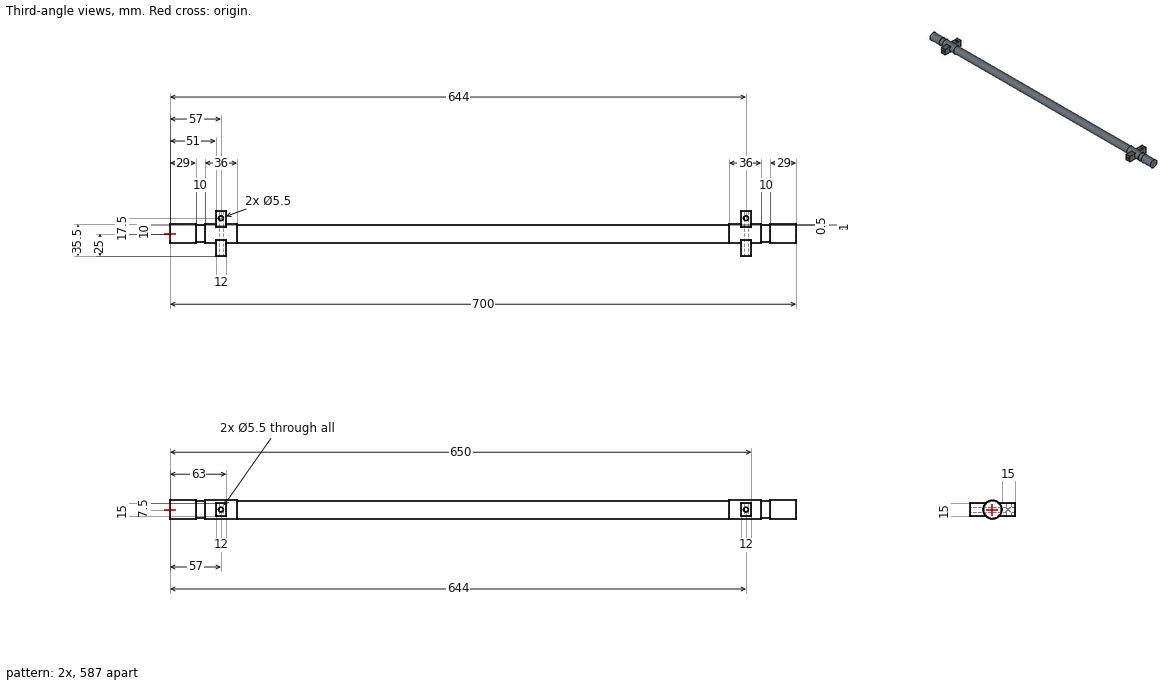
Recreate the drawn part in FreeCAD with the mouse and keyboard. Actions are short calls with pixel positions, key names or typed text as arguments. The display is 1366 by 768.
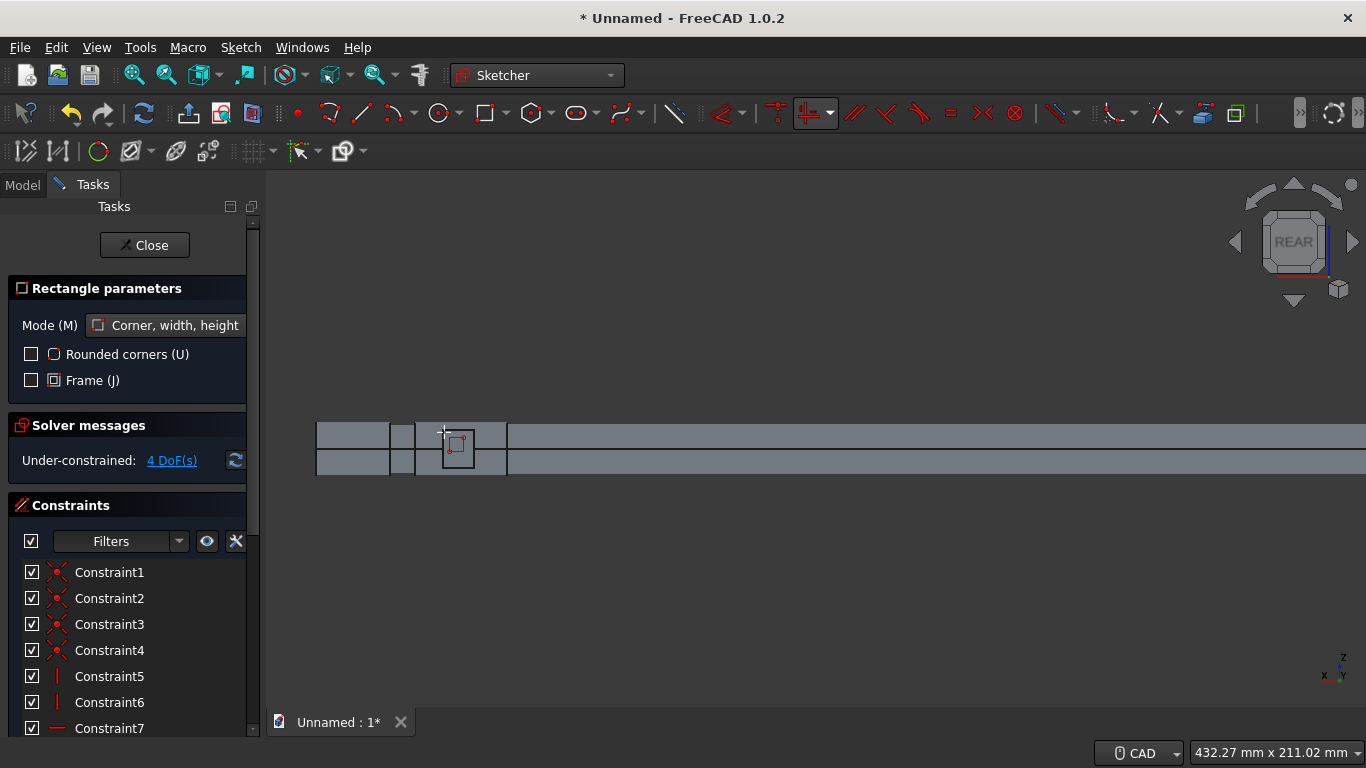
click(443, 430)
click(474, 468)
key(Escape)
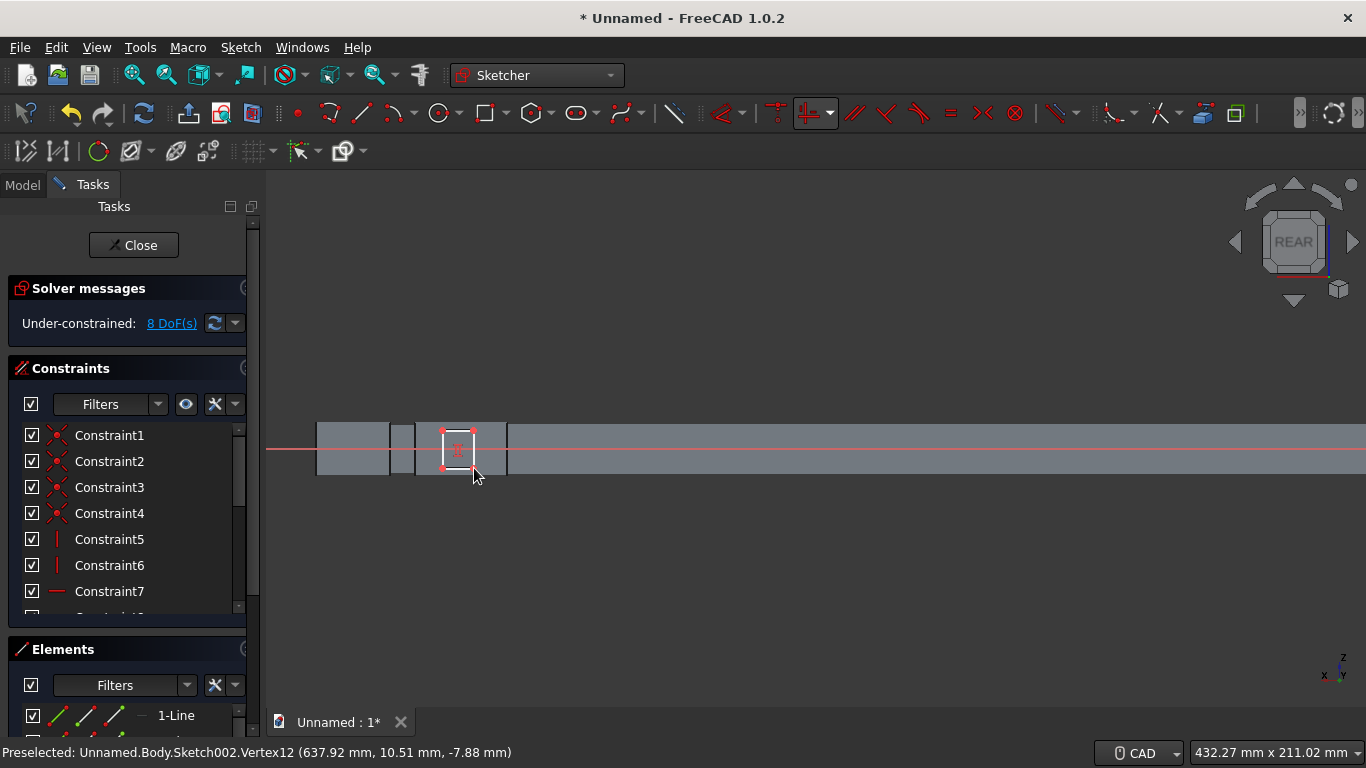
click(722, 114)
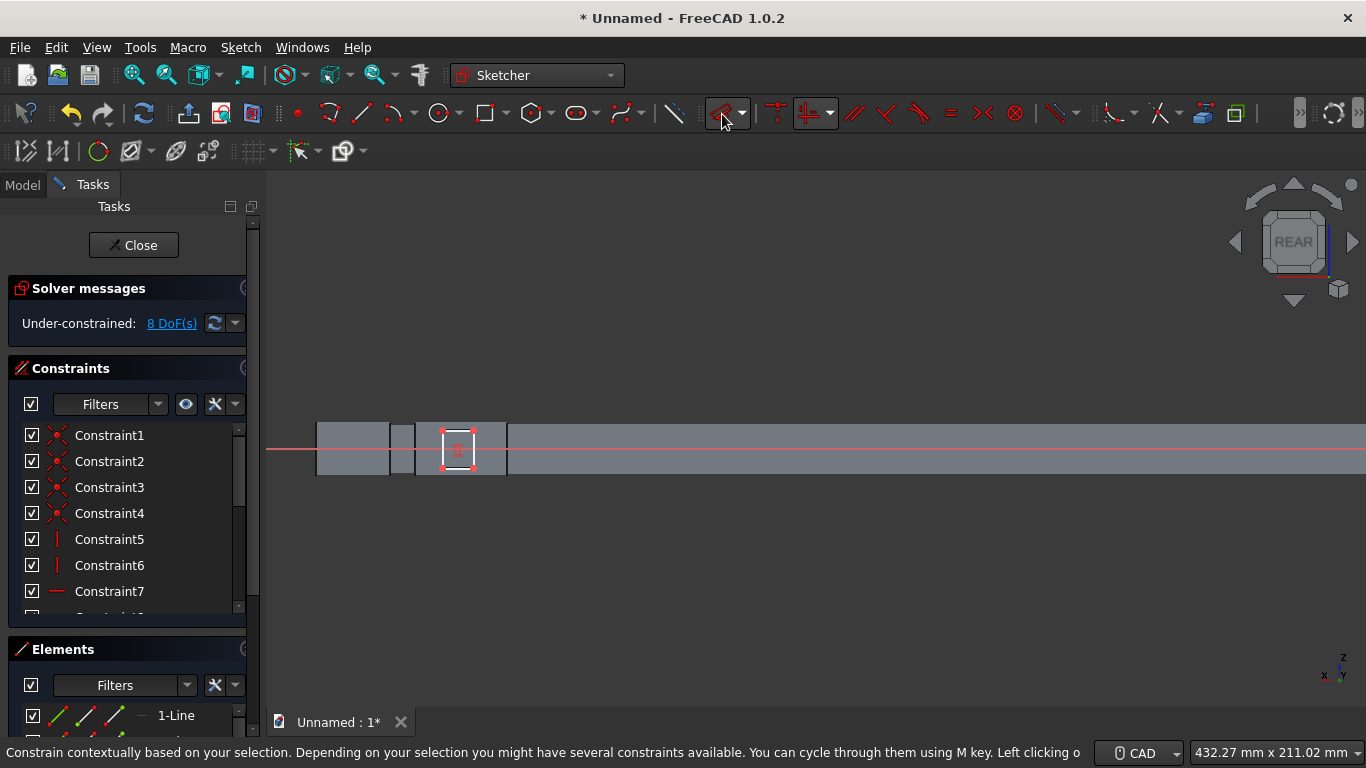
scroll(443, 432, down, 5)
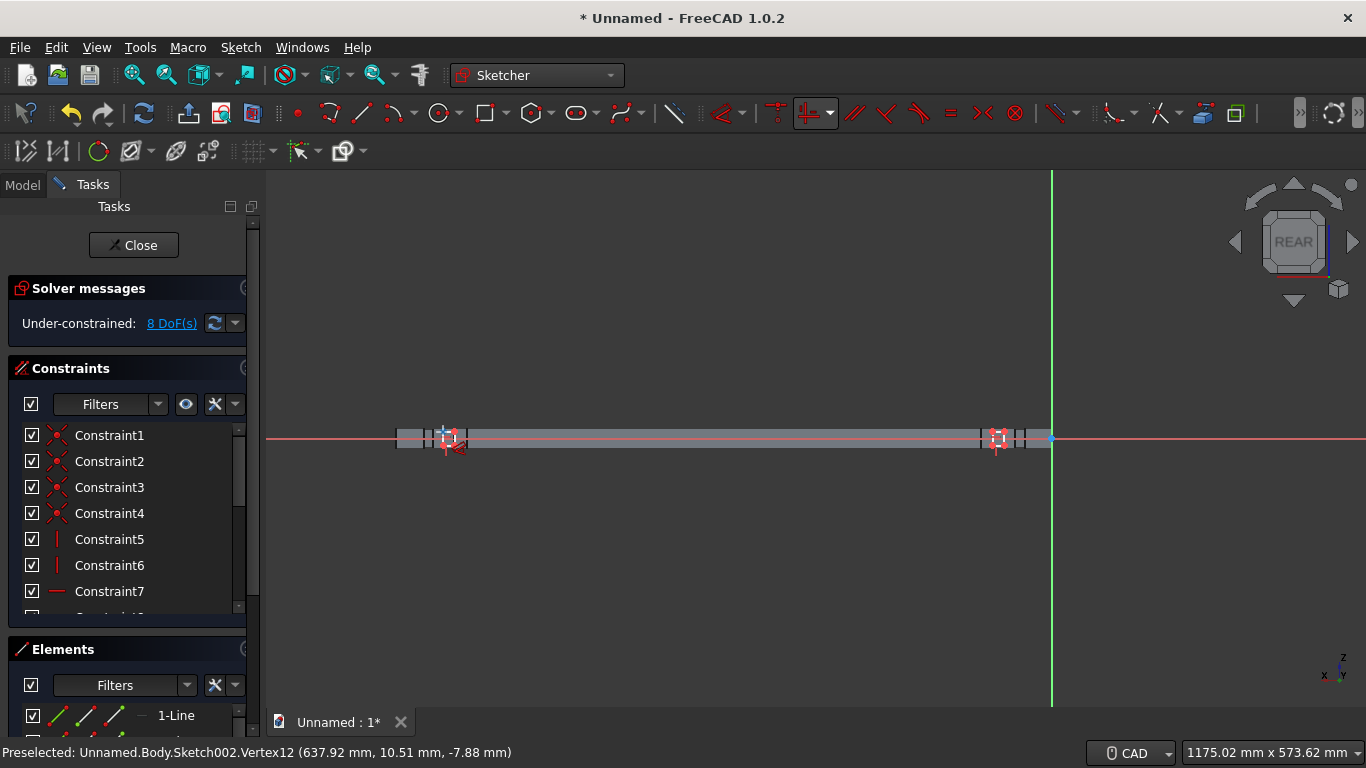
scroll(993, 438, up, 6)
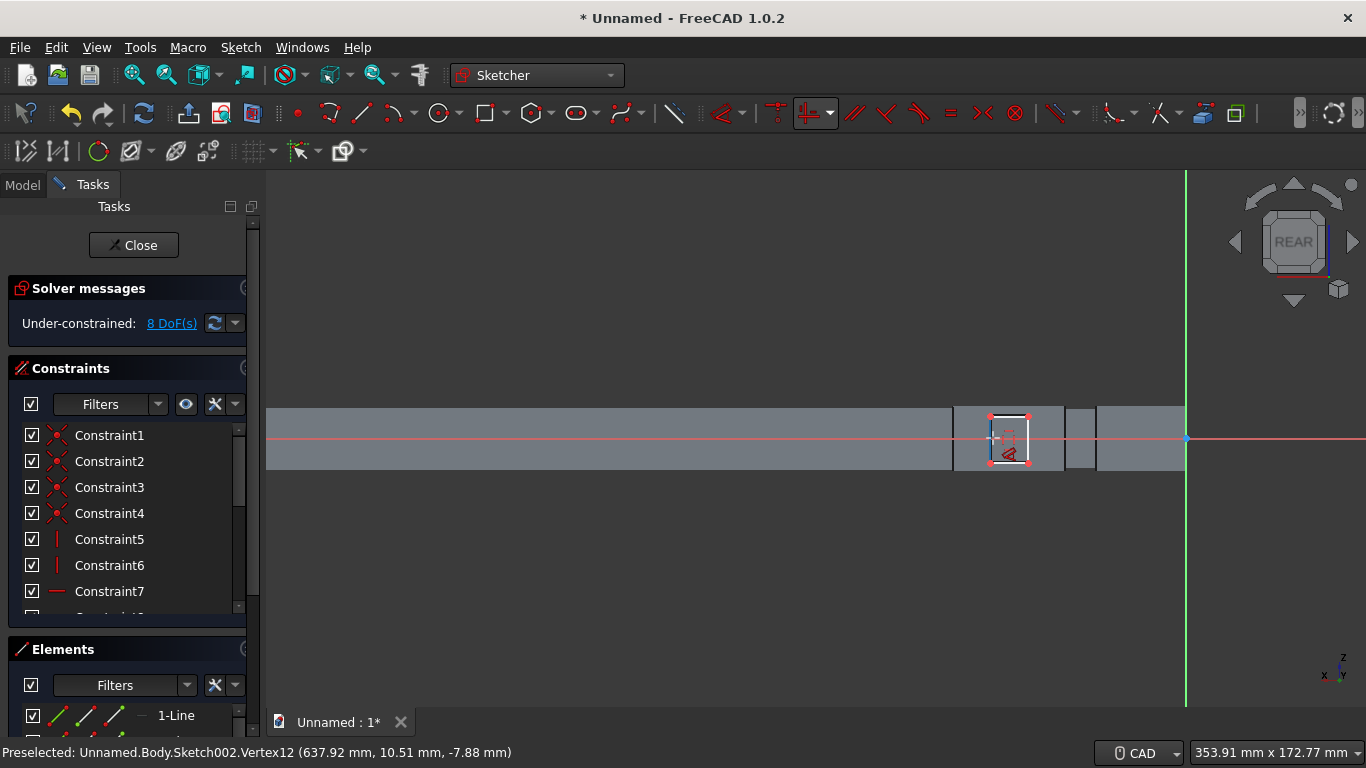
click(990, 435)
click(956, 424)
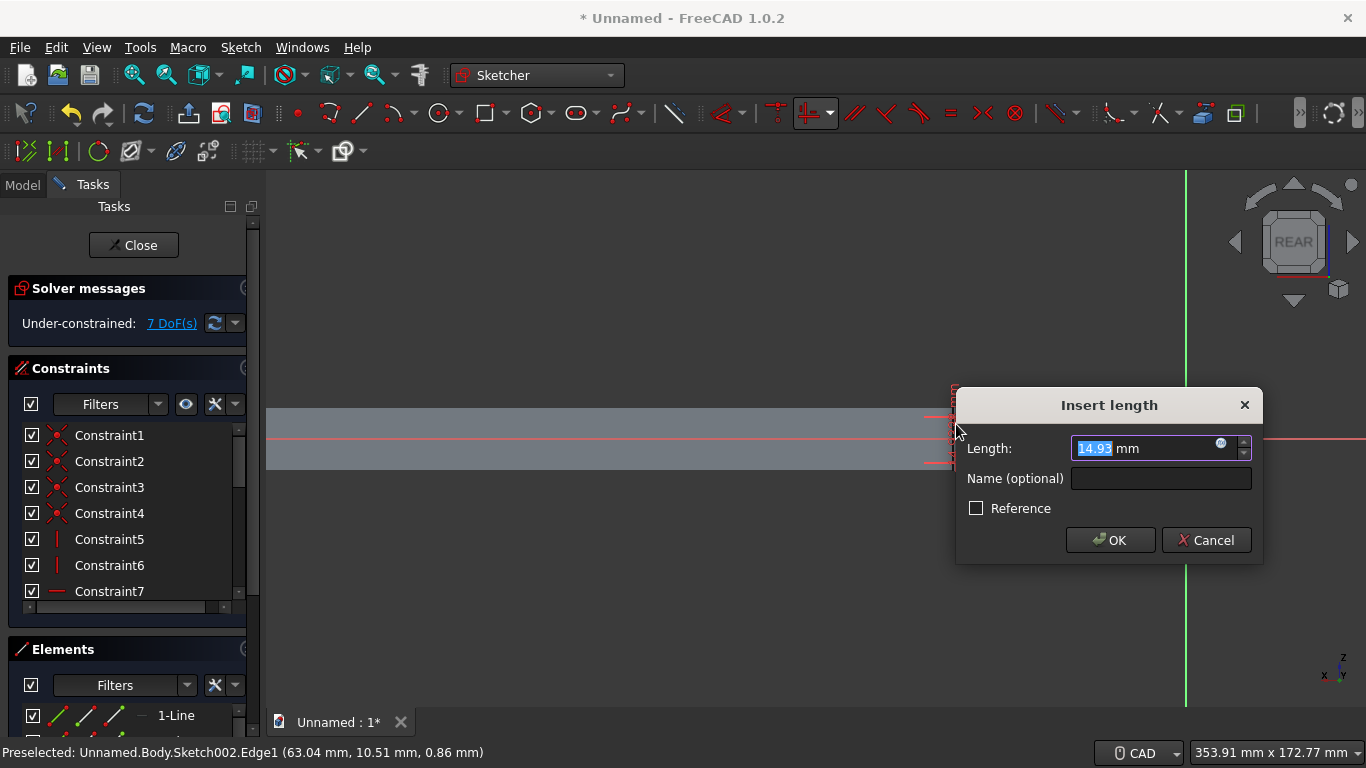
text(15)
key(Return)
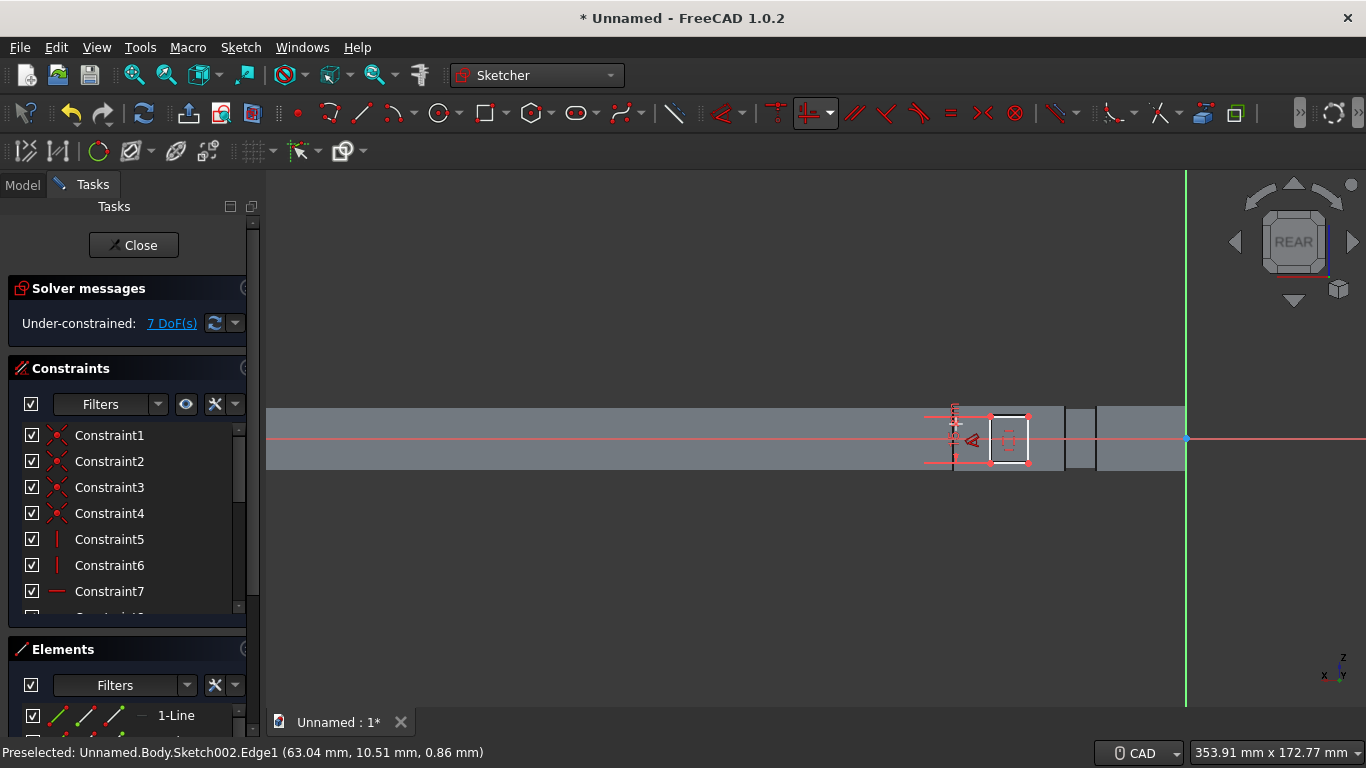
click(1002, 463)
click(1009, 497)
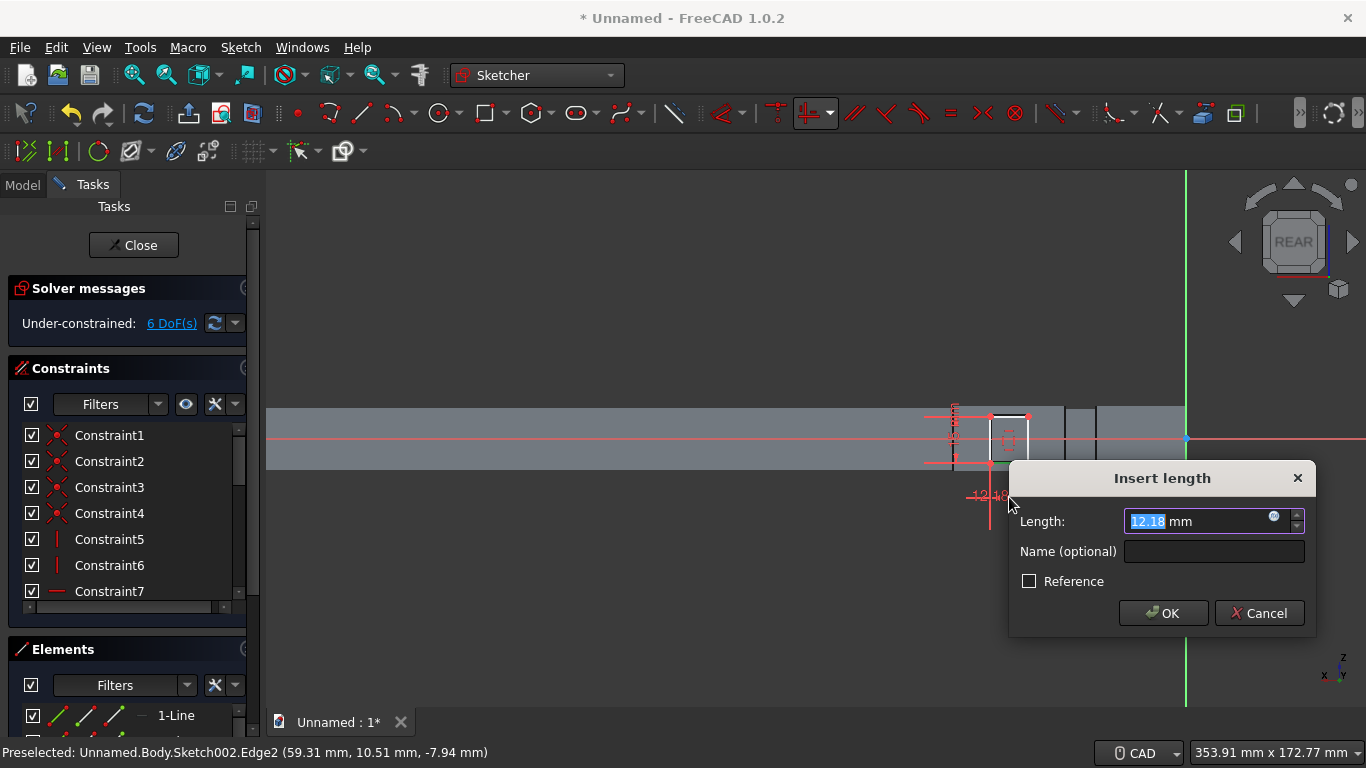
text(12)
key(Return)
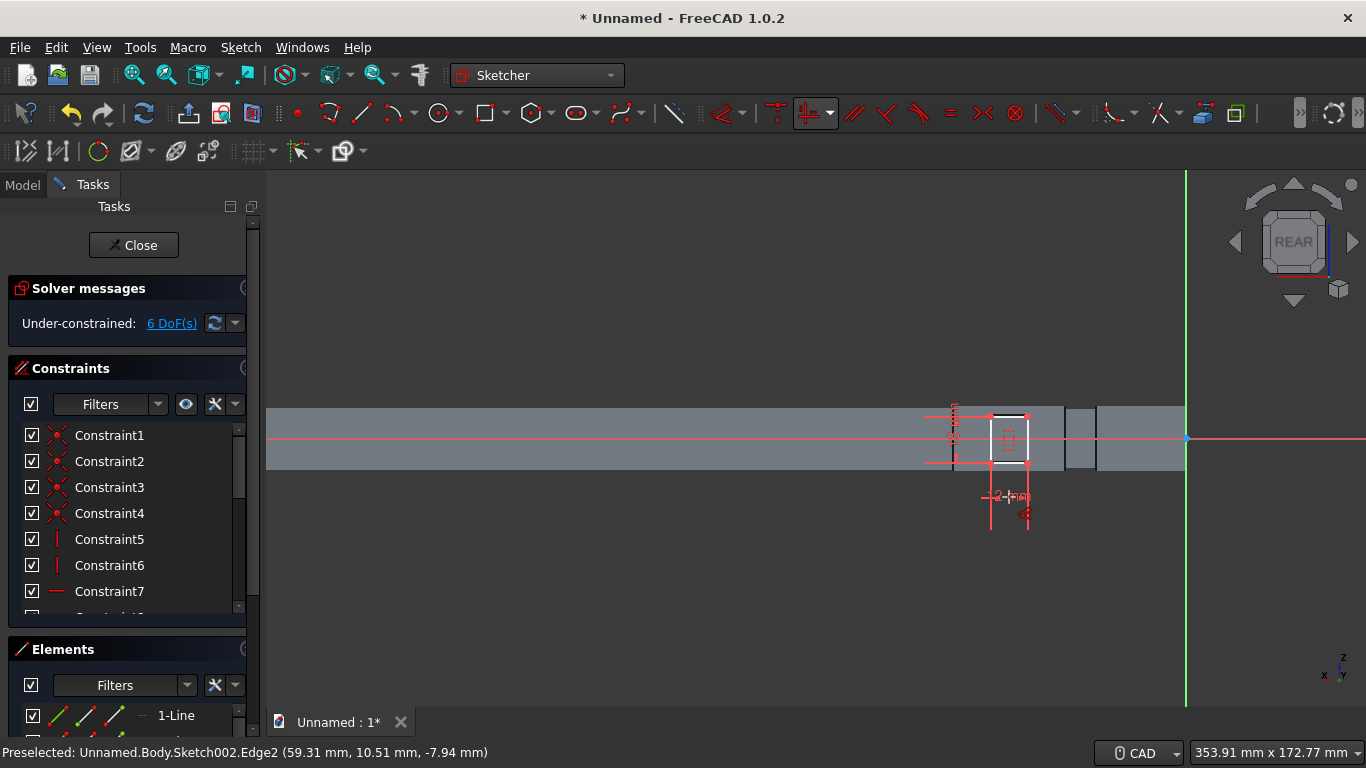
scroll(994, 438, down, 6)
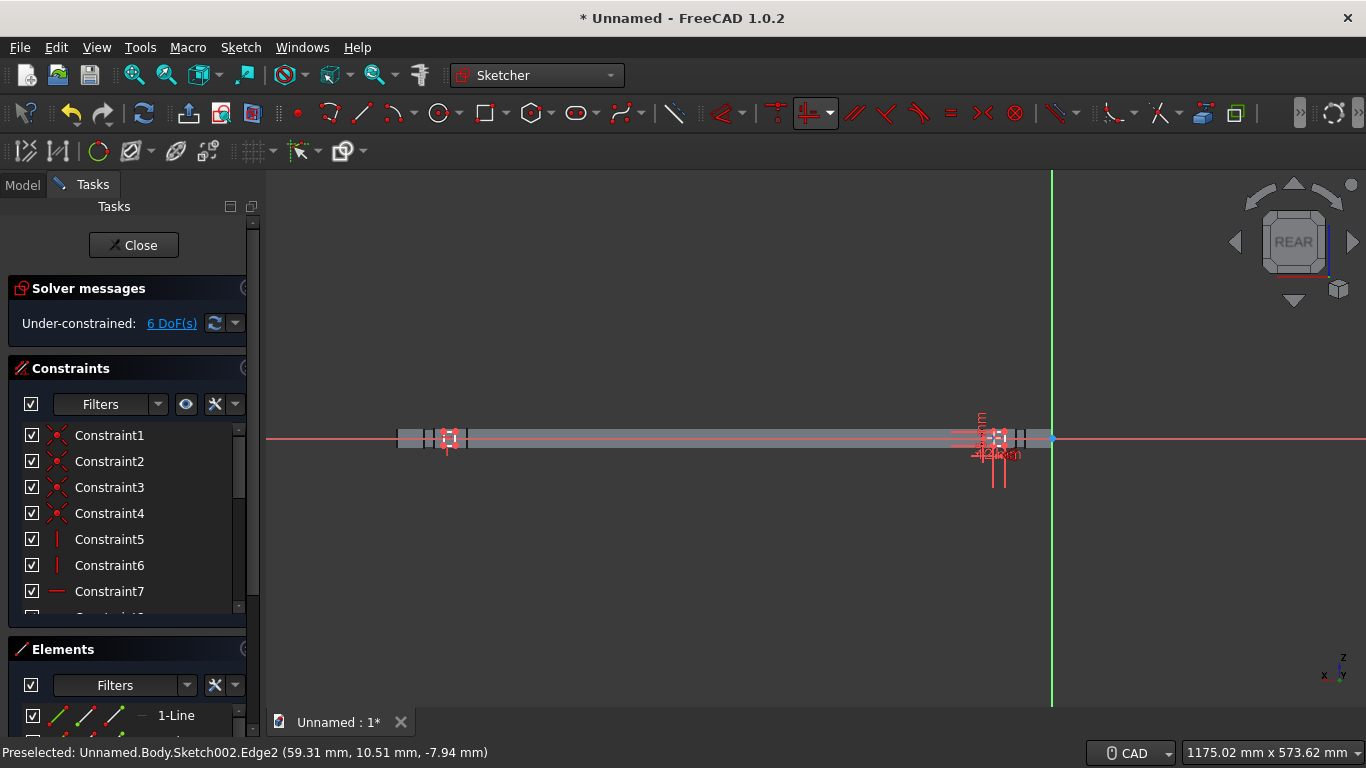
scroll(444, 442, up, 8)